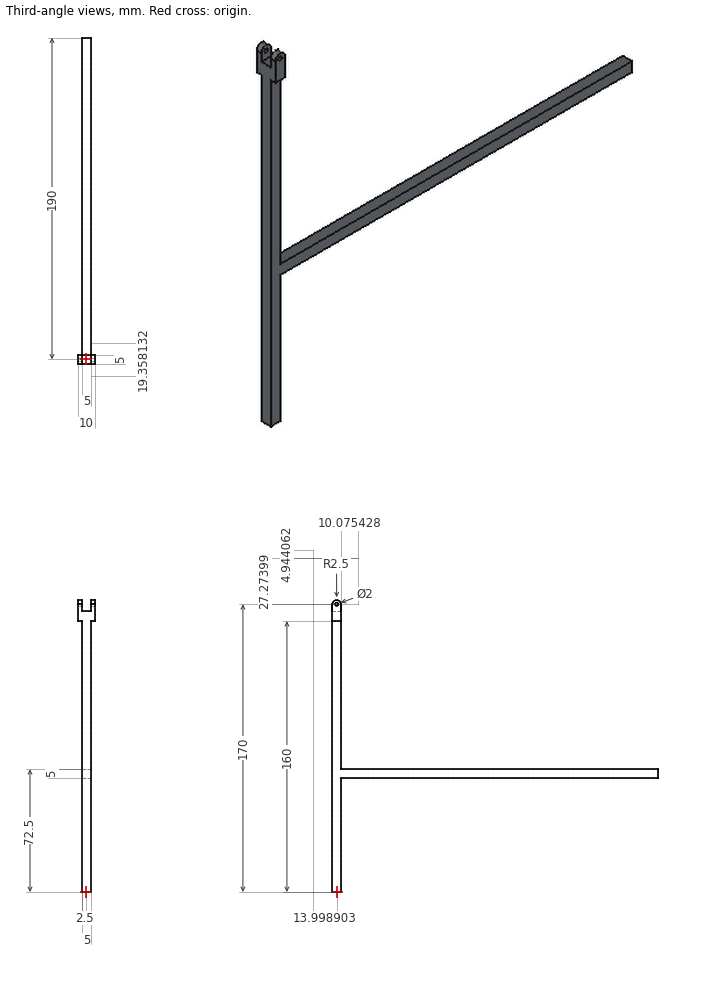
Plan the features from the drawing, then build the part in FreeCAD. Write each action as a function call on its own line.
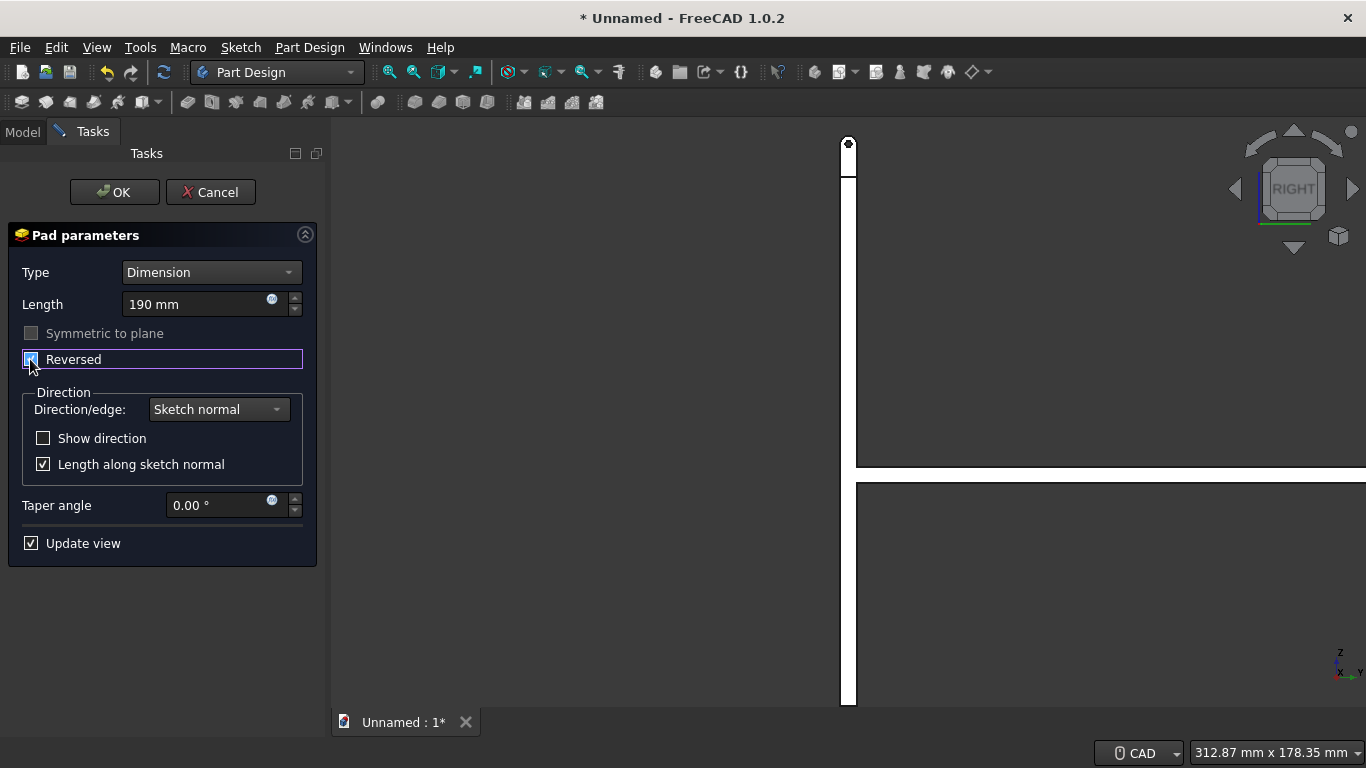
click(115, 192)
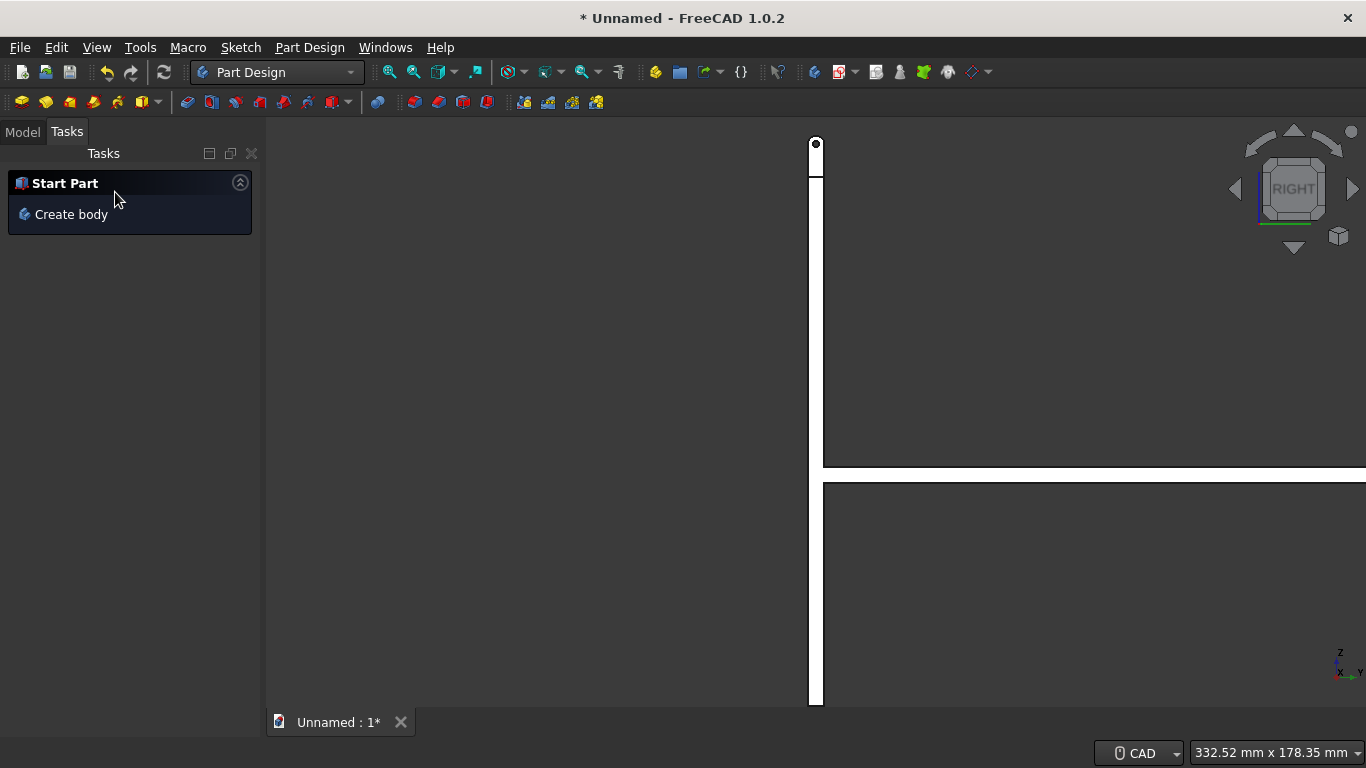
key(0)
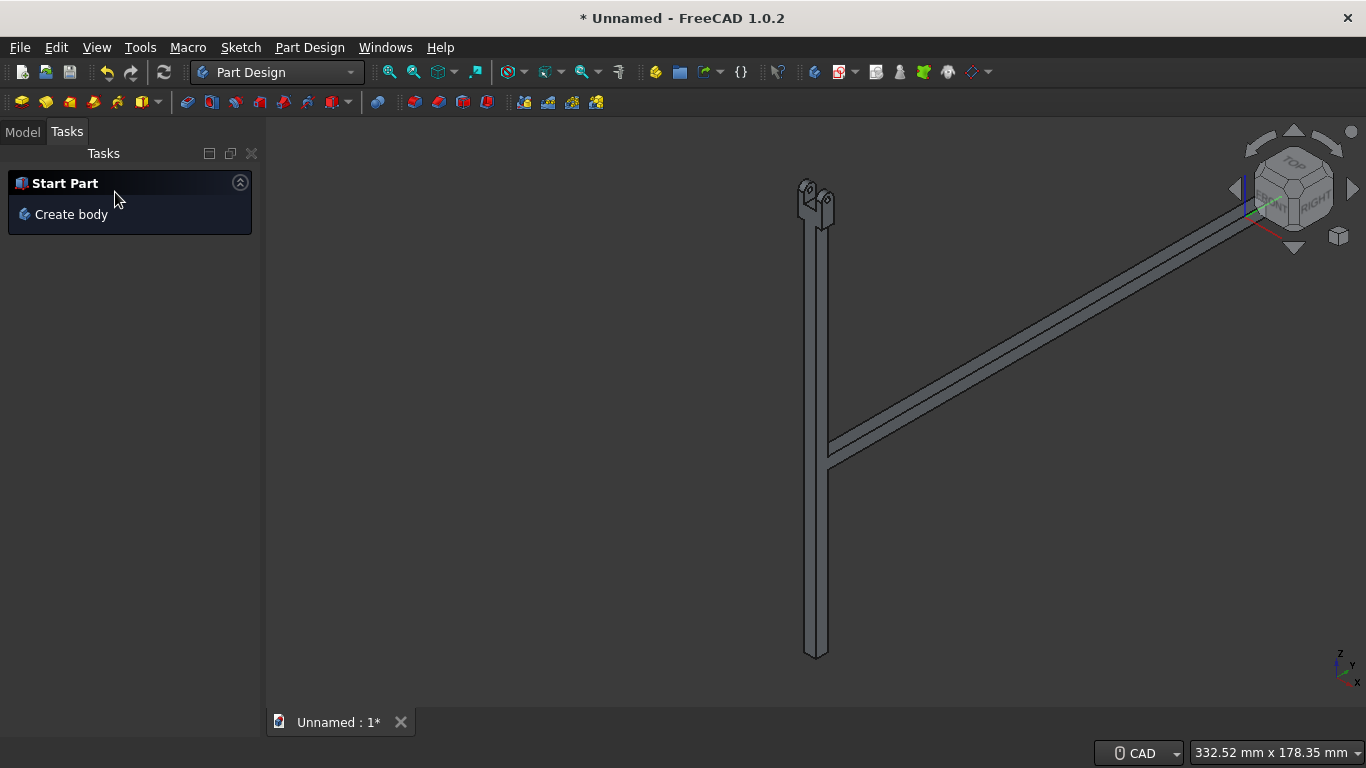
click(390, 72)